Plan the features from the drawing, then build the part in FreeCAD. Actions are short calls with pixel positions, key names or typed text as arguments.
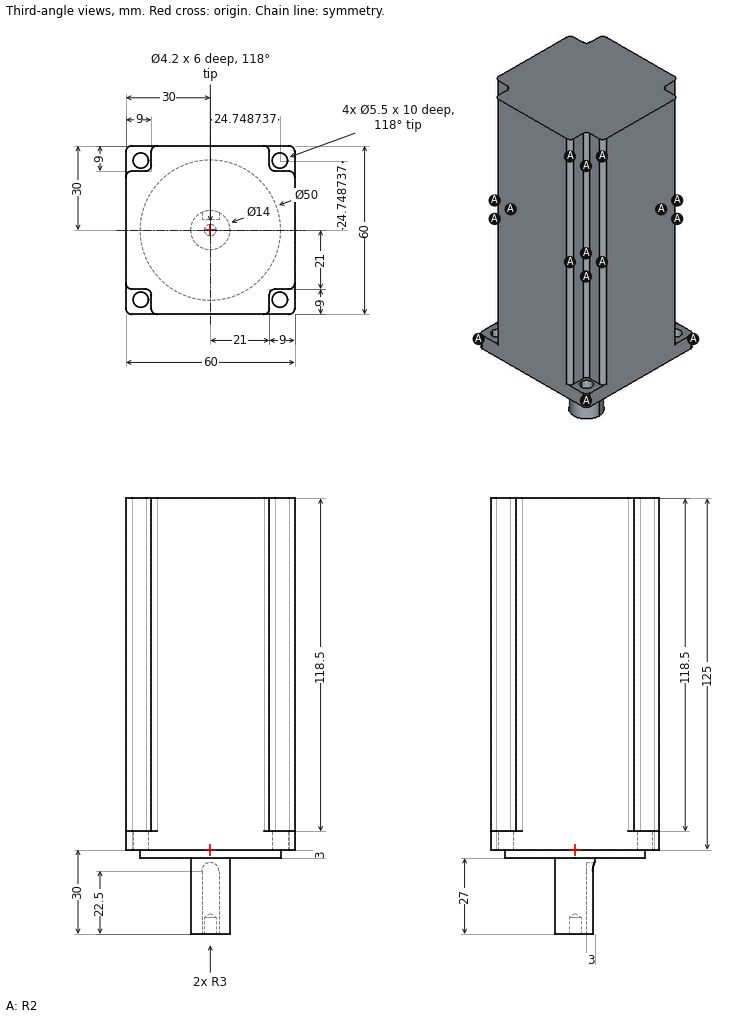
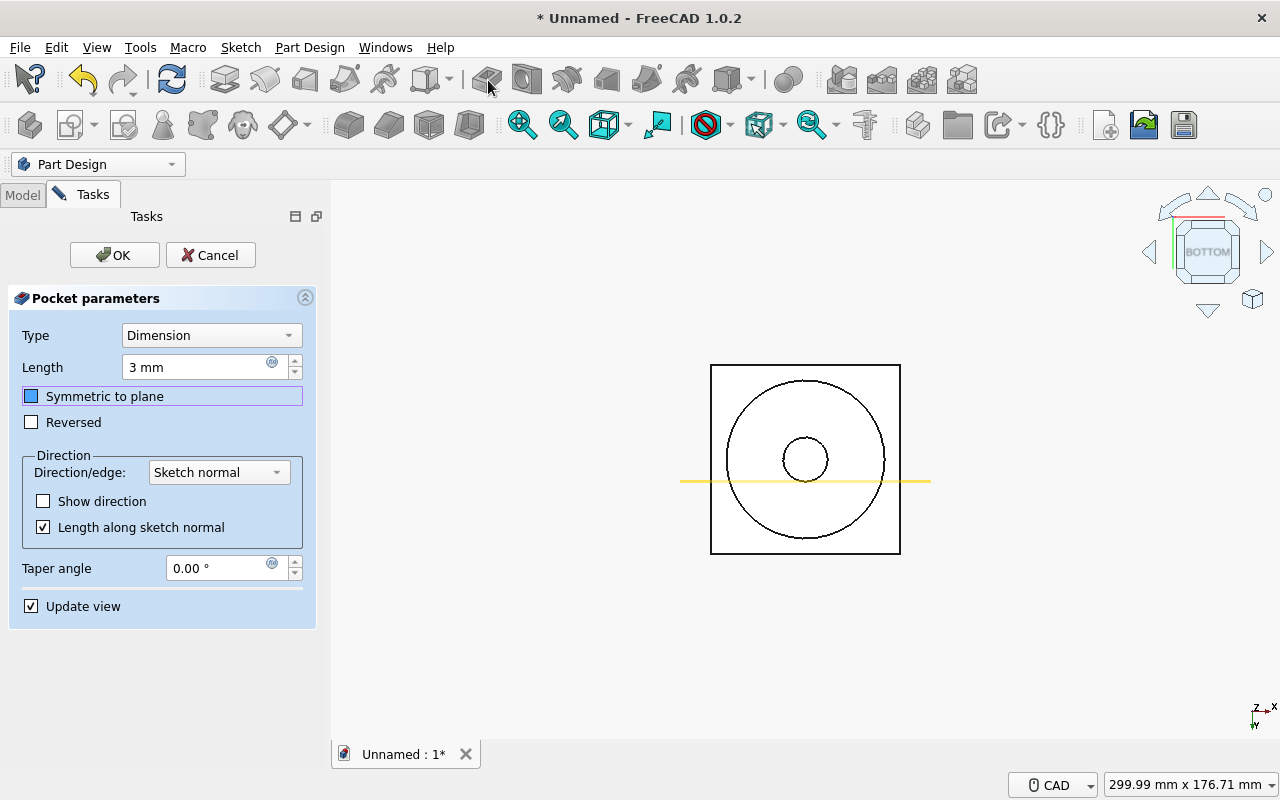
click(30, 422)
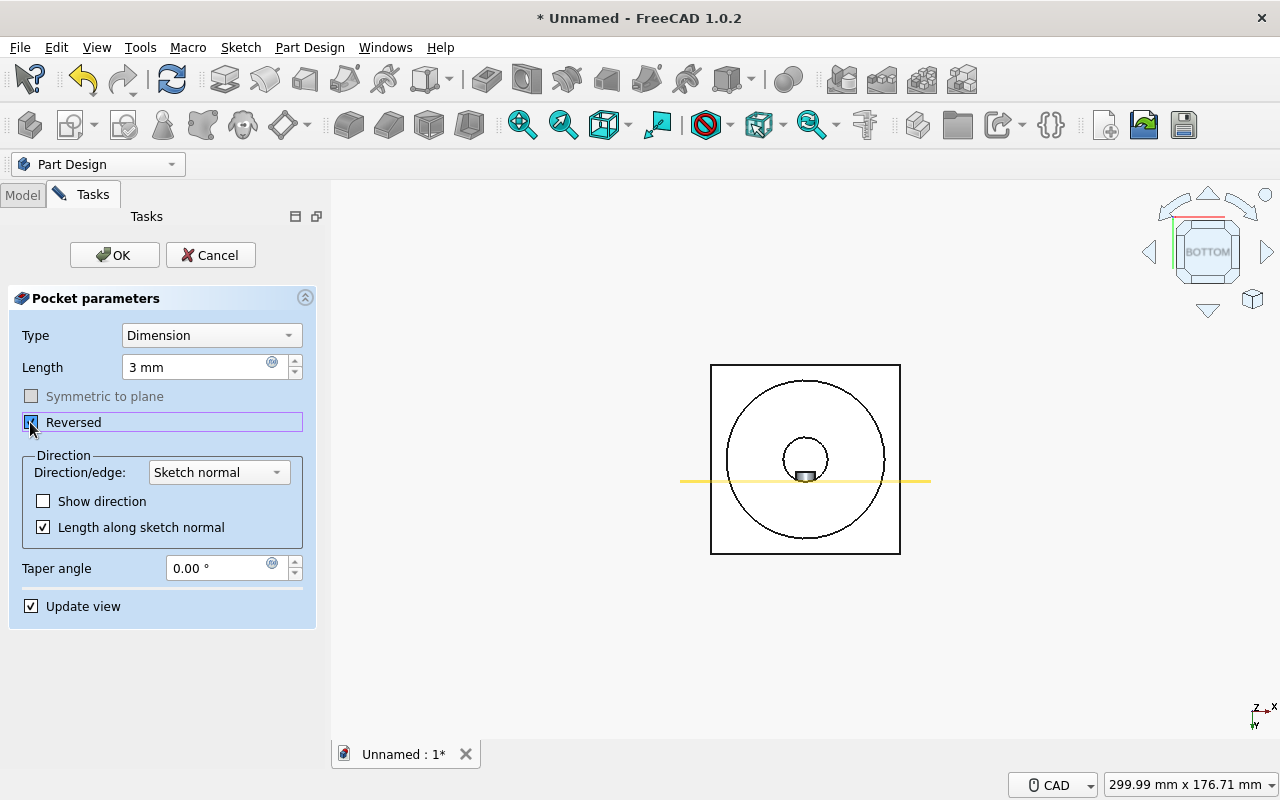
click(115, 255)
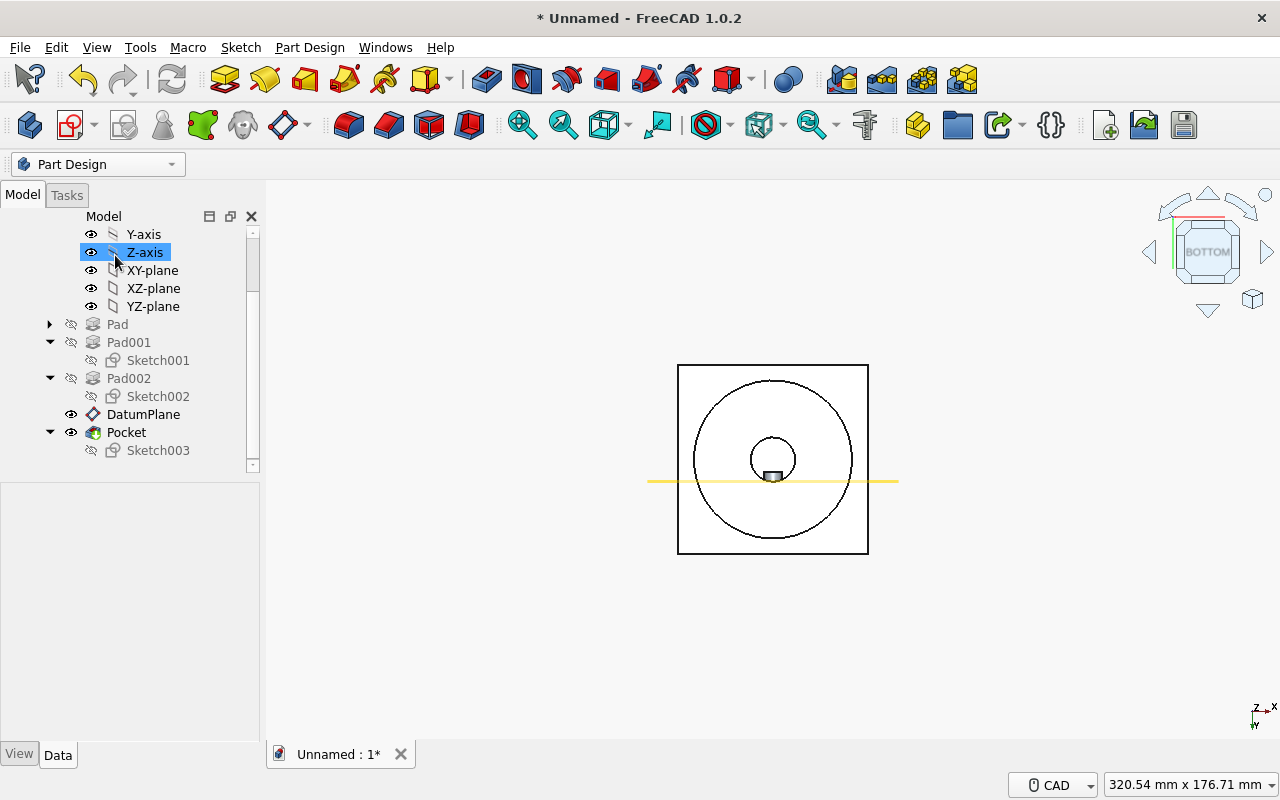
click(116, 414)
key(space)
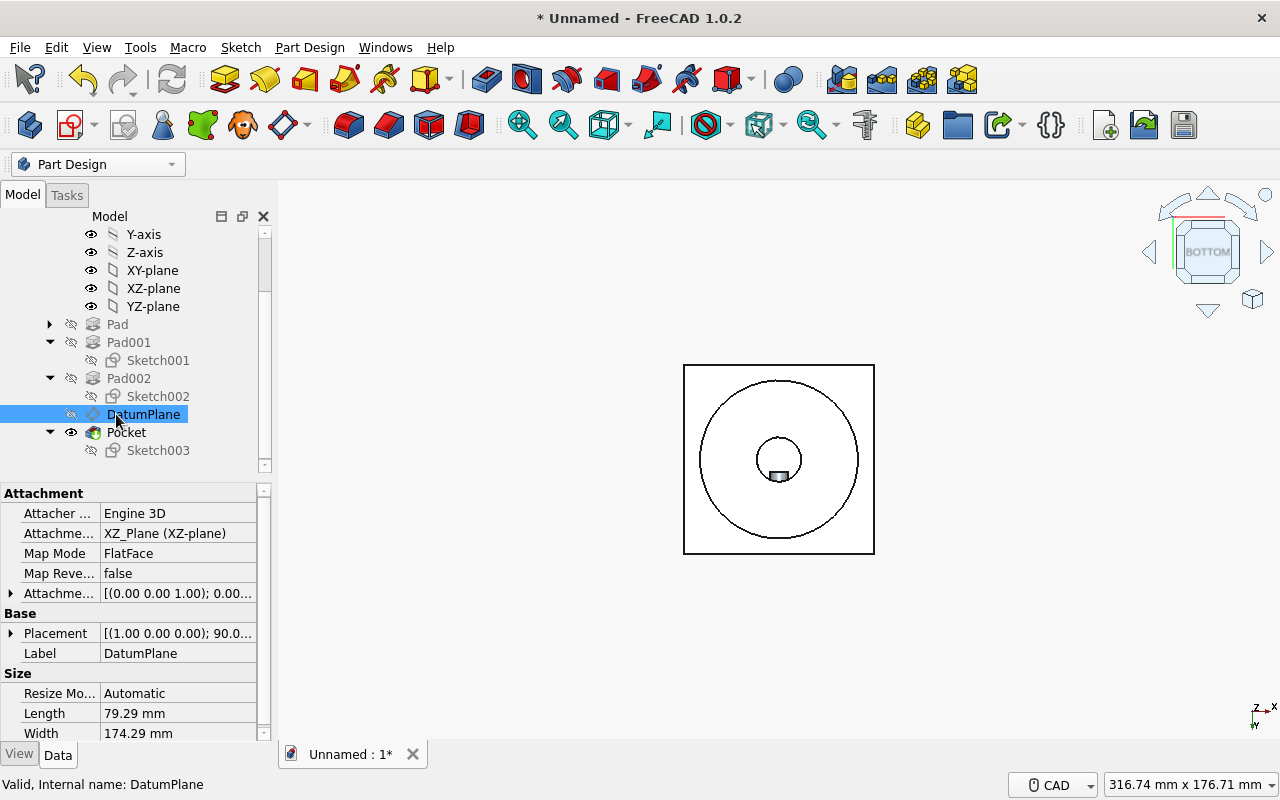
click(524, 126)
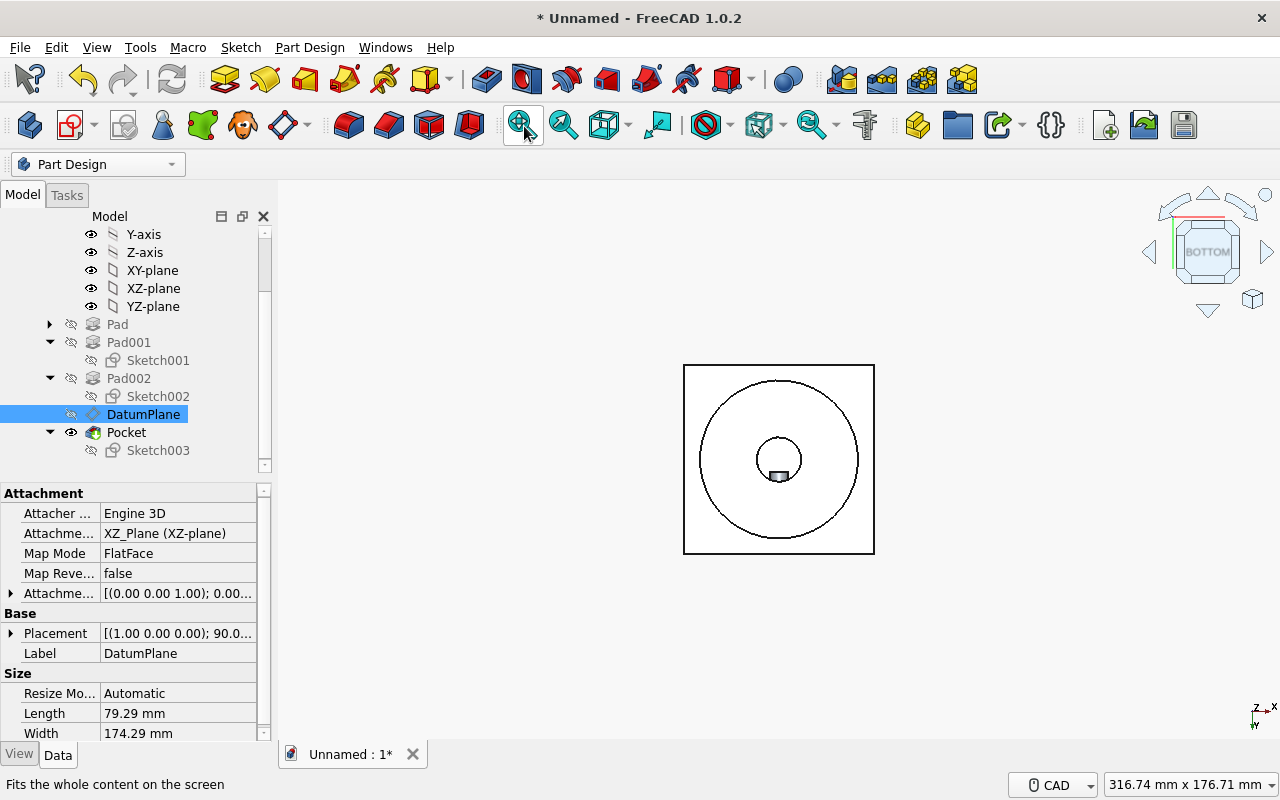
click(779, 451)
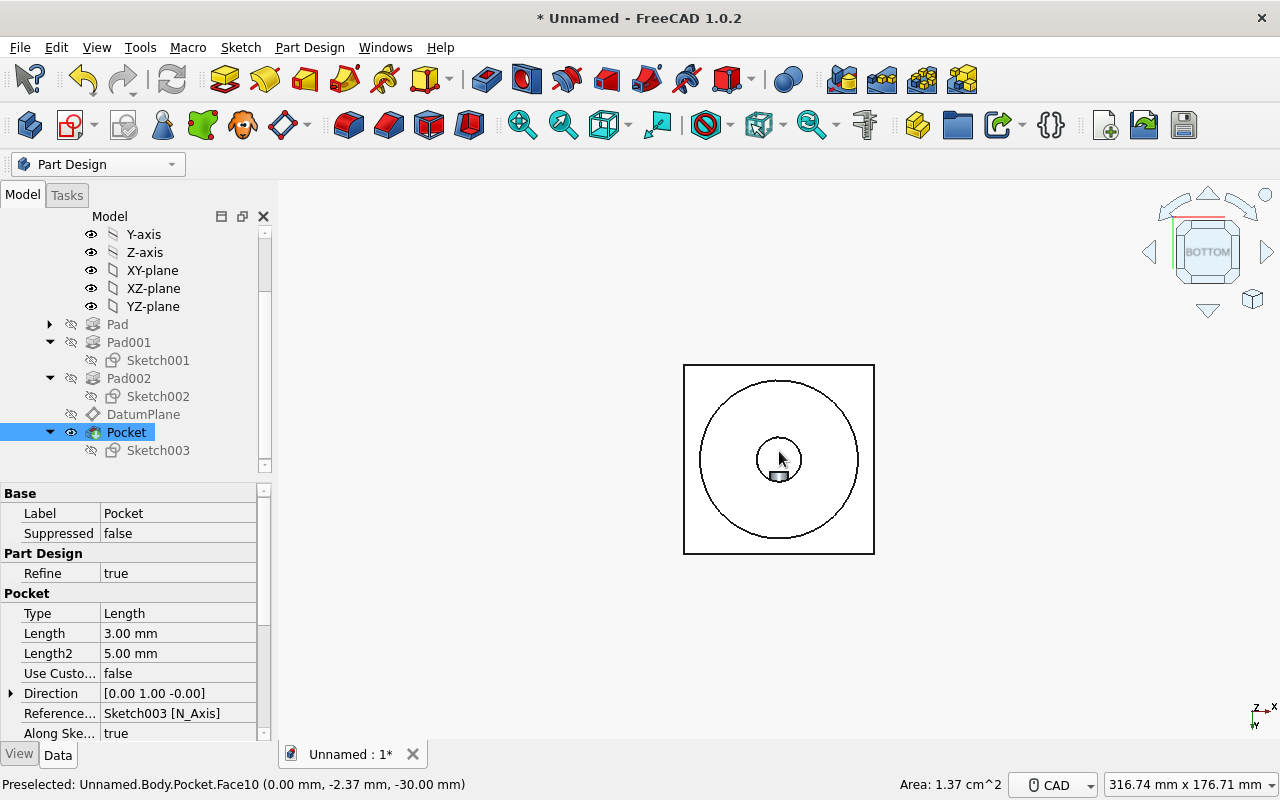
click(70, 126)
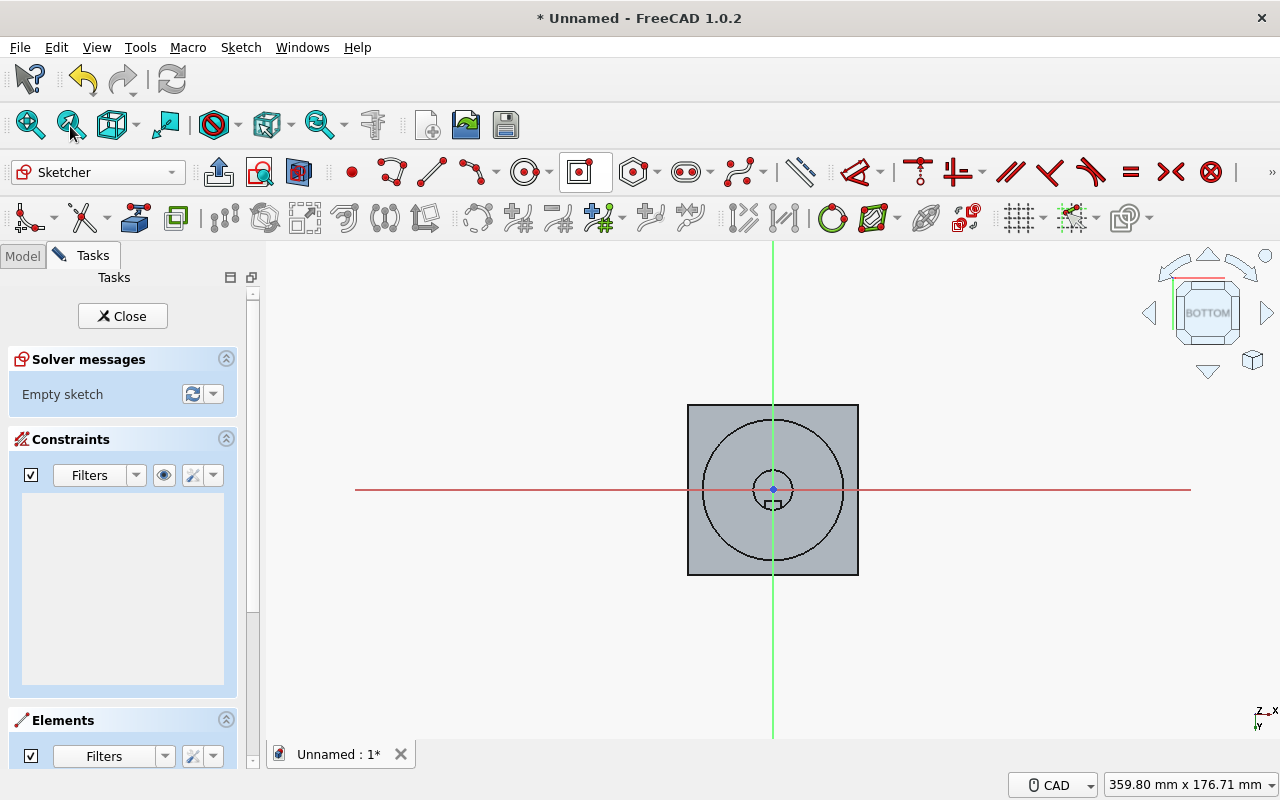
scroll(777, 490, up, 15)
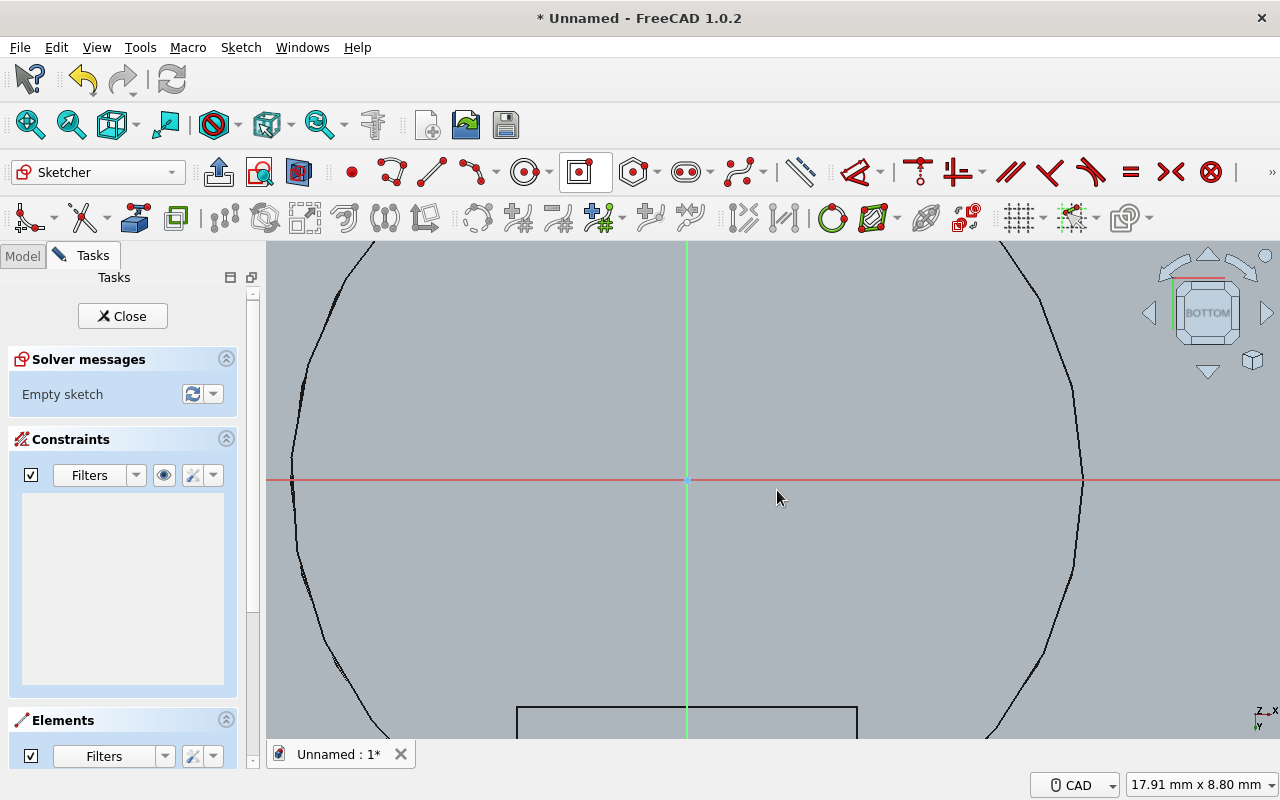
click(526, 172)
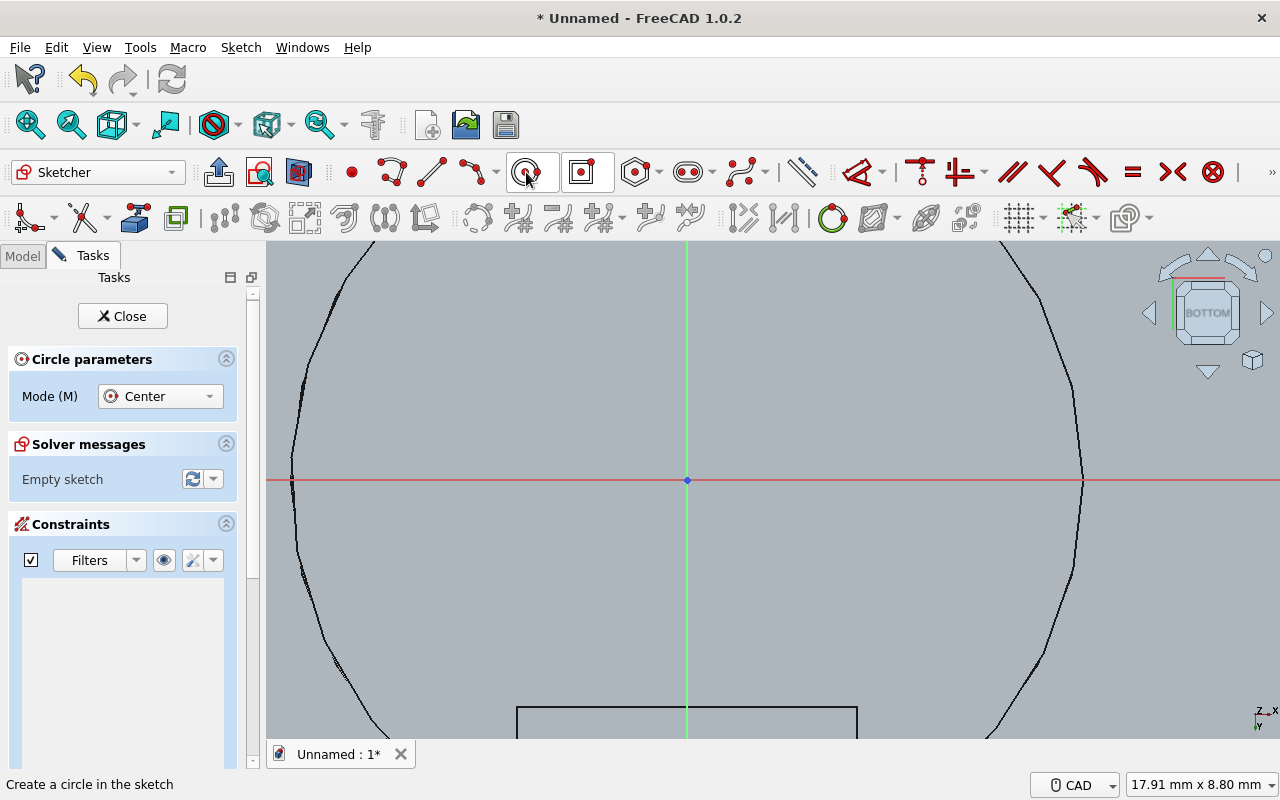
click(687, 480)
move(771, 396)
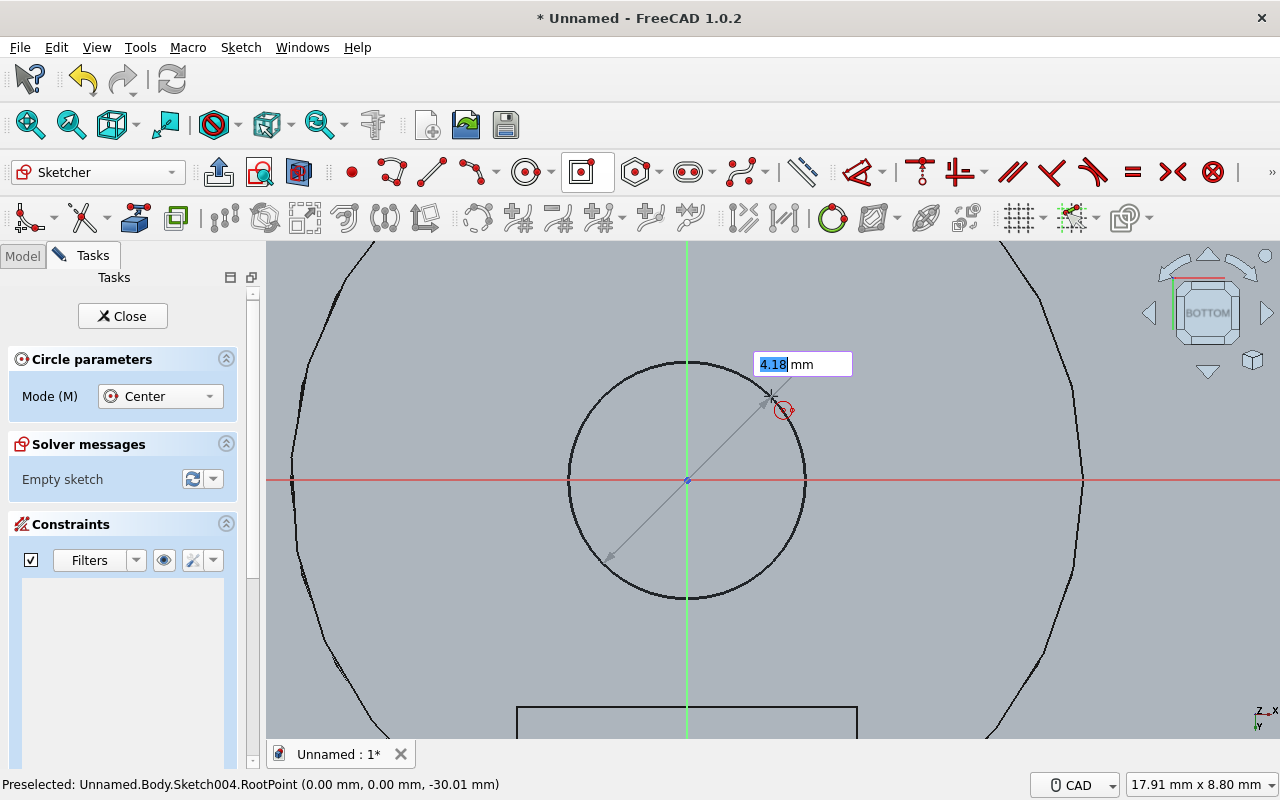
text(4.2)
key(Return)
key(Escape)